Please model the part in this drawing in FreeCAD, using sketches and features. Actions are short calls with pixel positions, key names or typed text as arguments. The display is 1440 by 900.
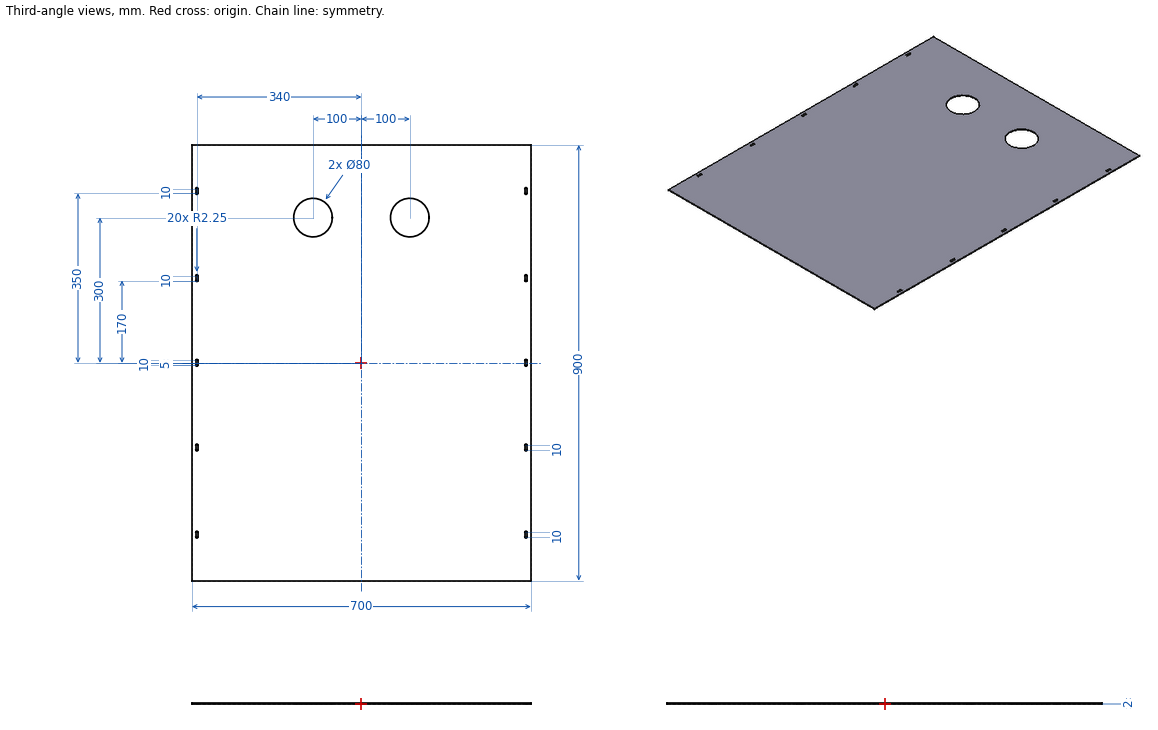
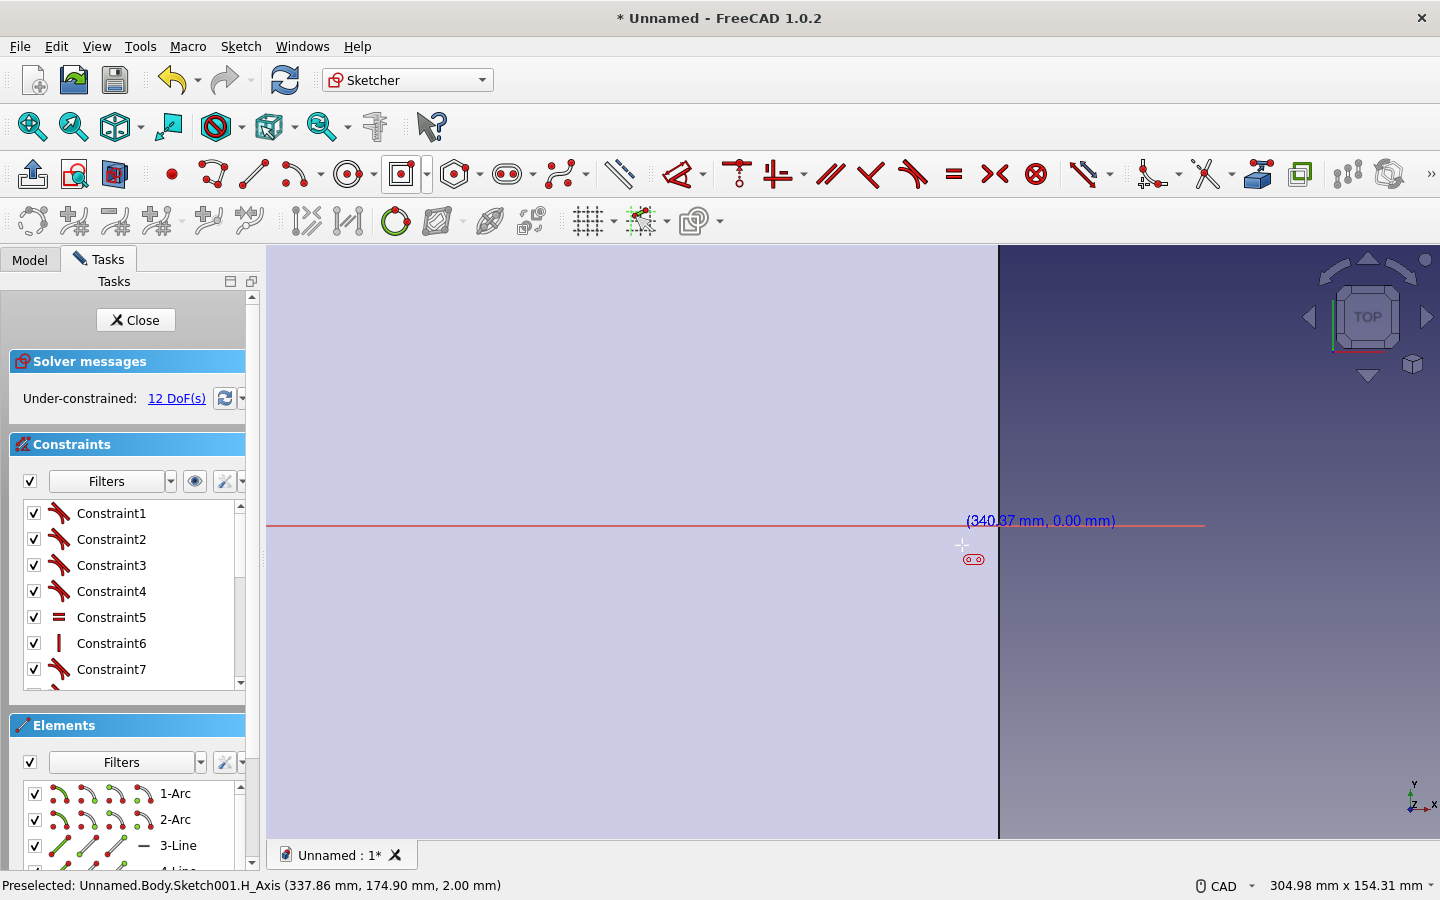
click(961, 545)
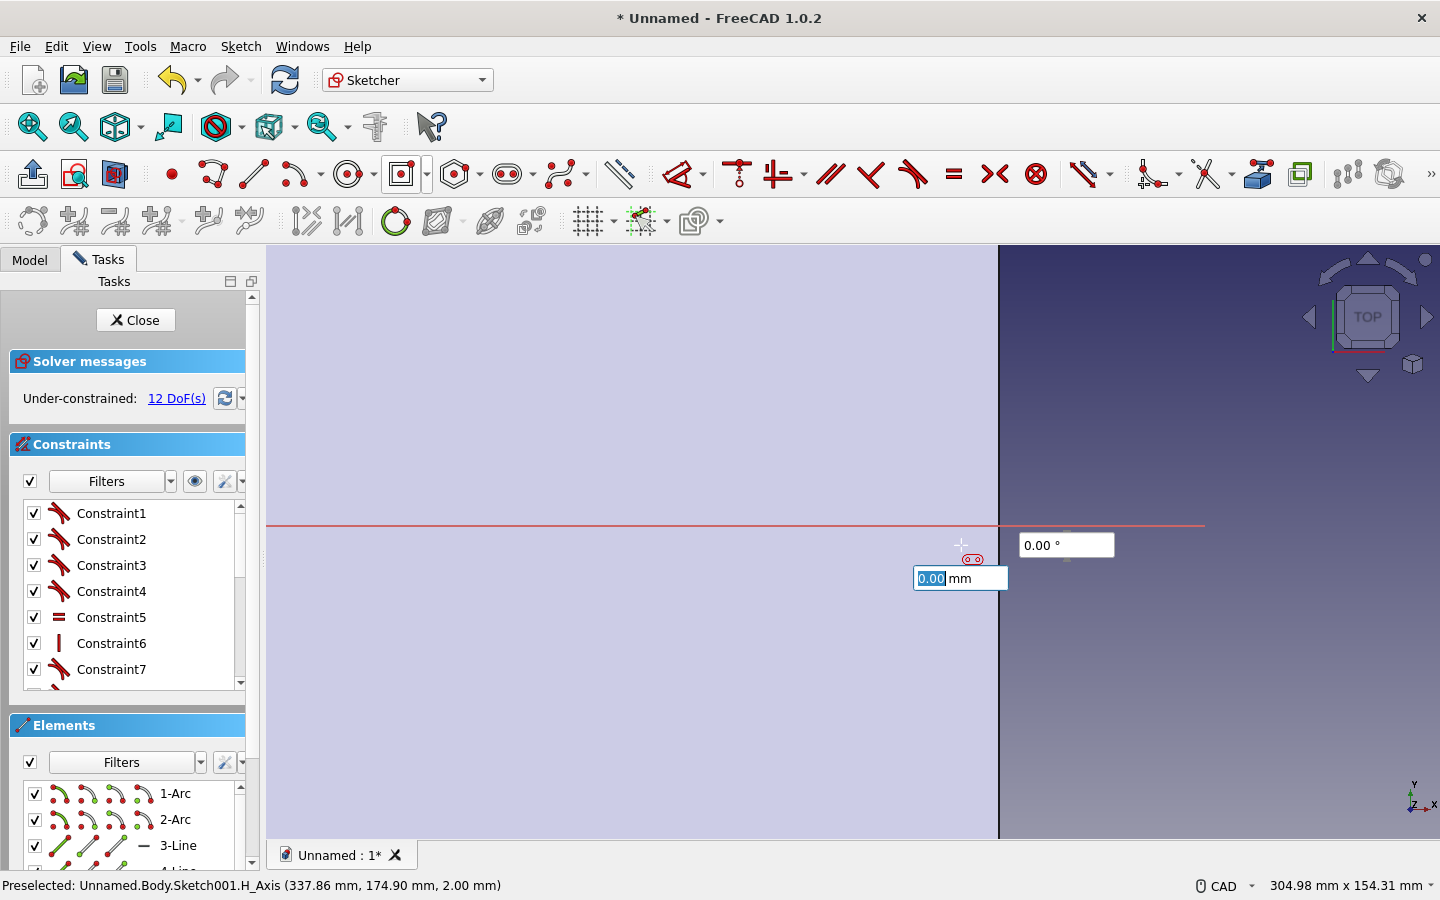
click(961, 506)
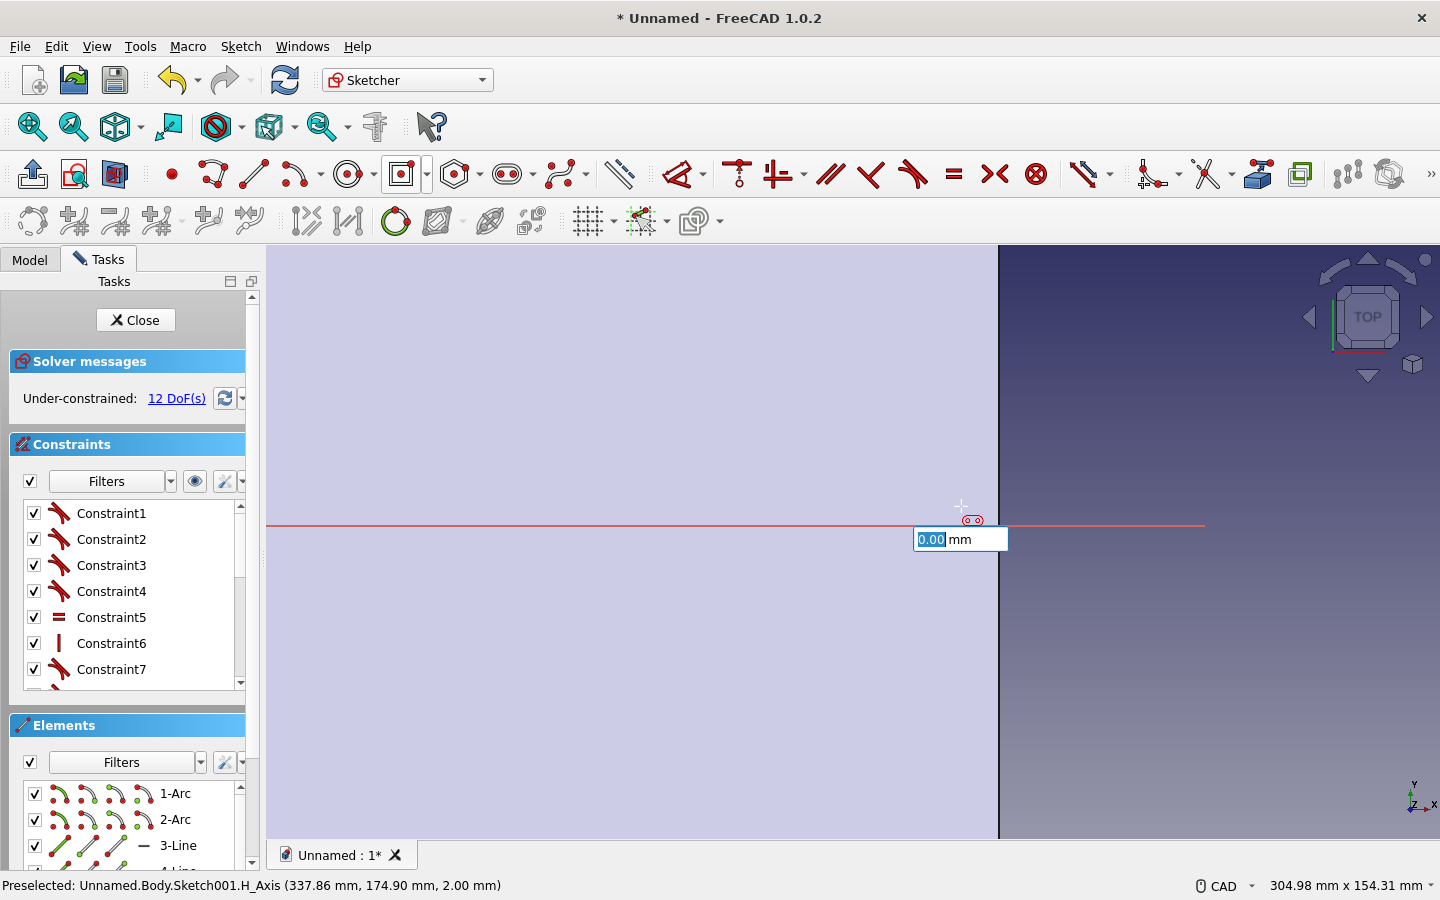
scroll(970, 531, up, 6)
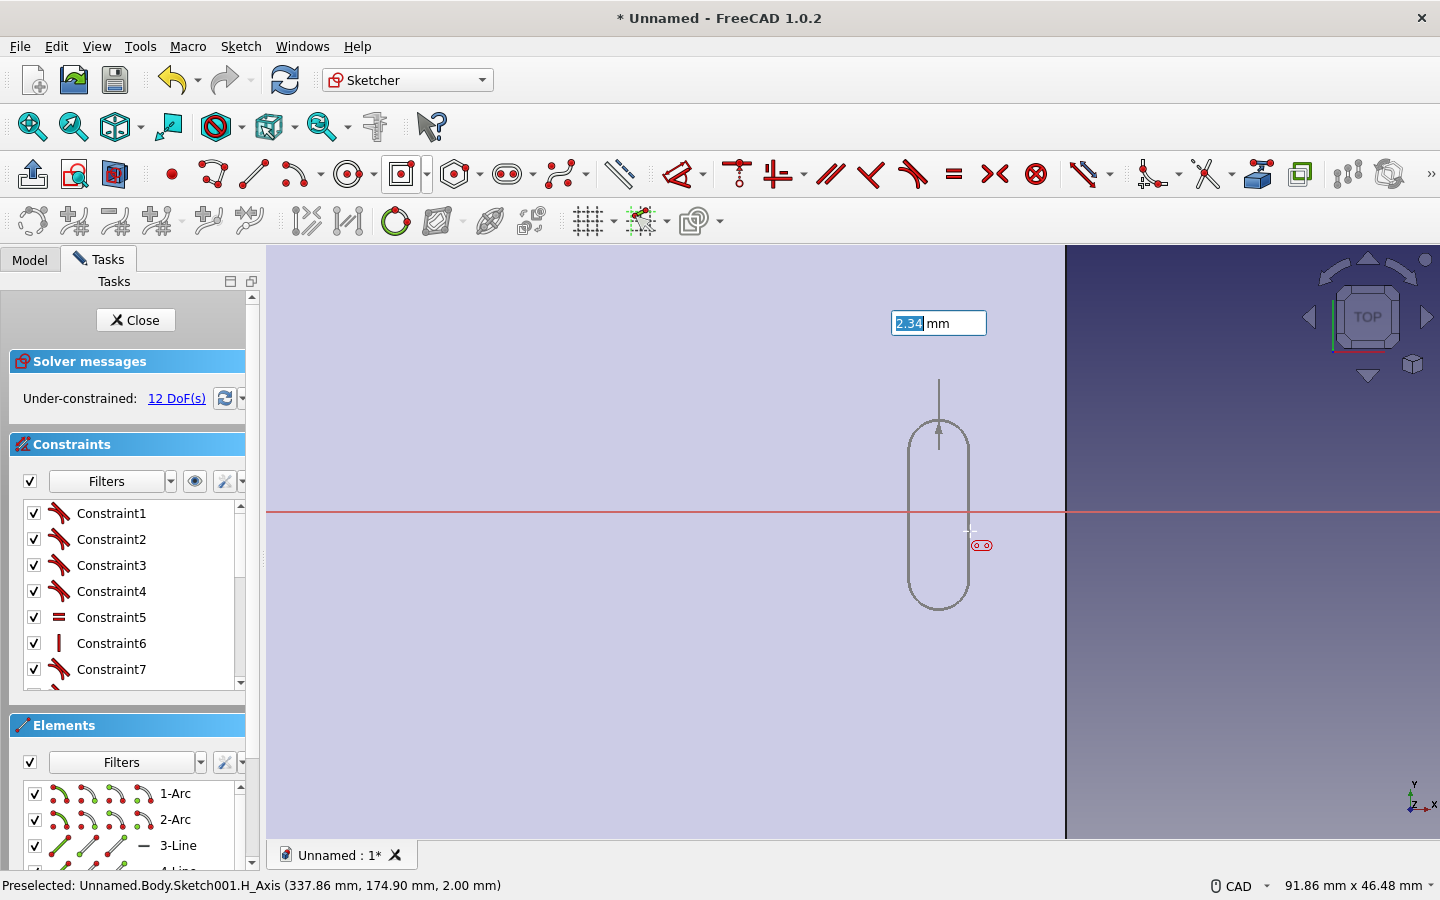
click(967, 531)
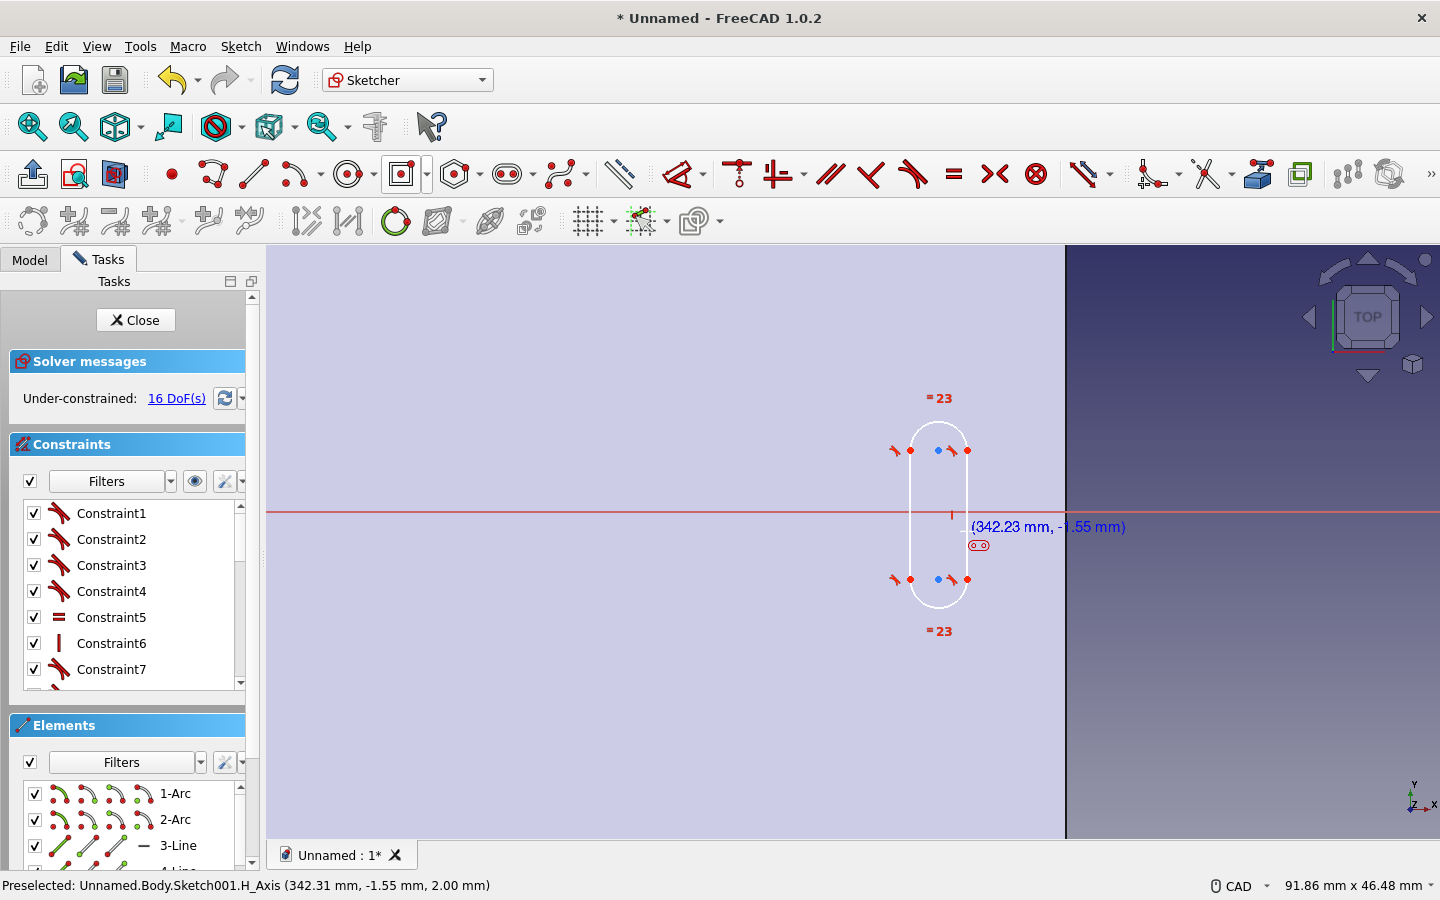
scroll(1004, 544, down, 15)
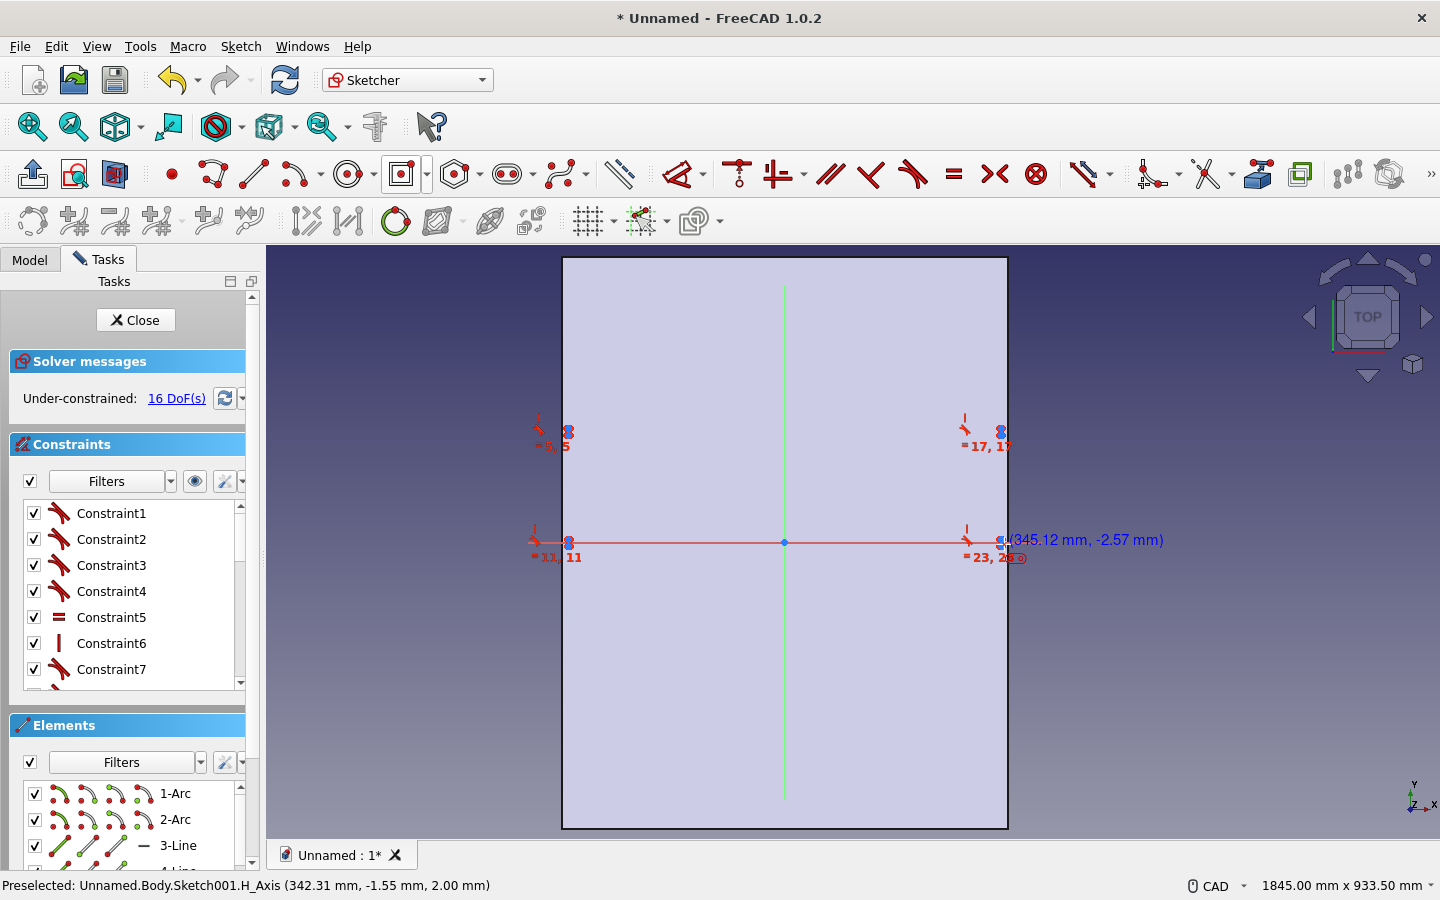
scroll(569, 320, up, 14)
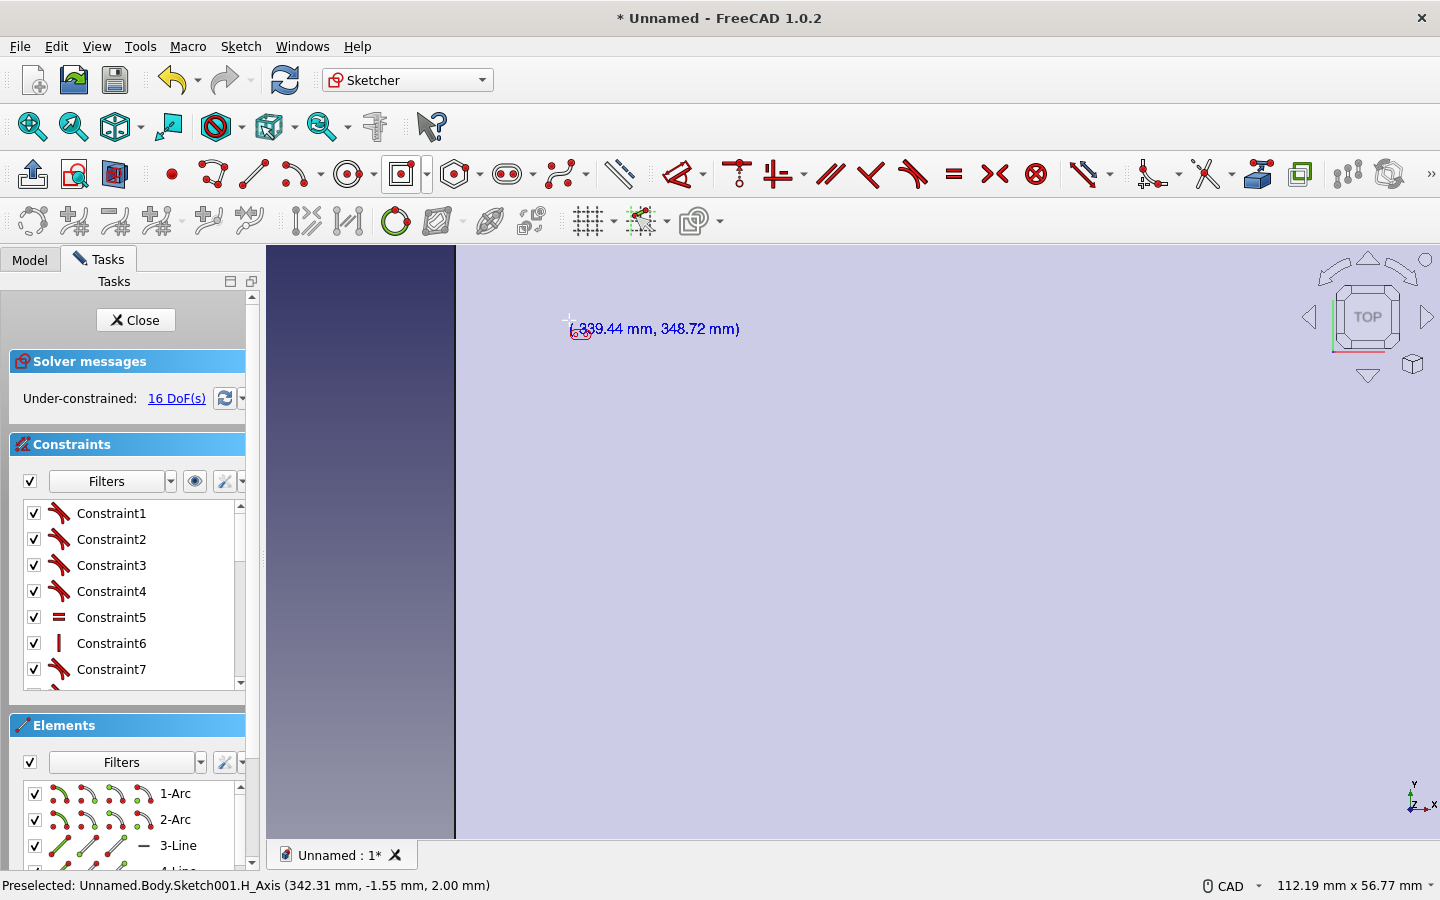
scroll(610, 362, down, 15)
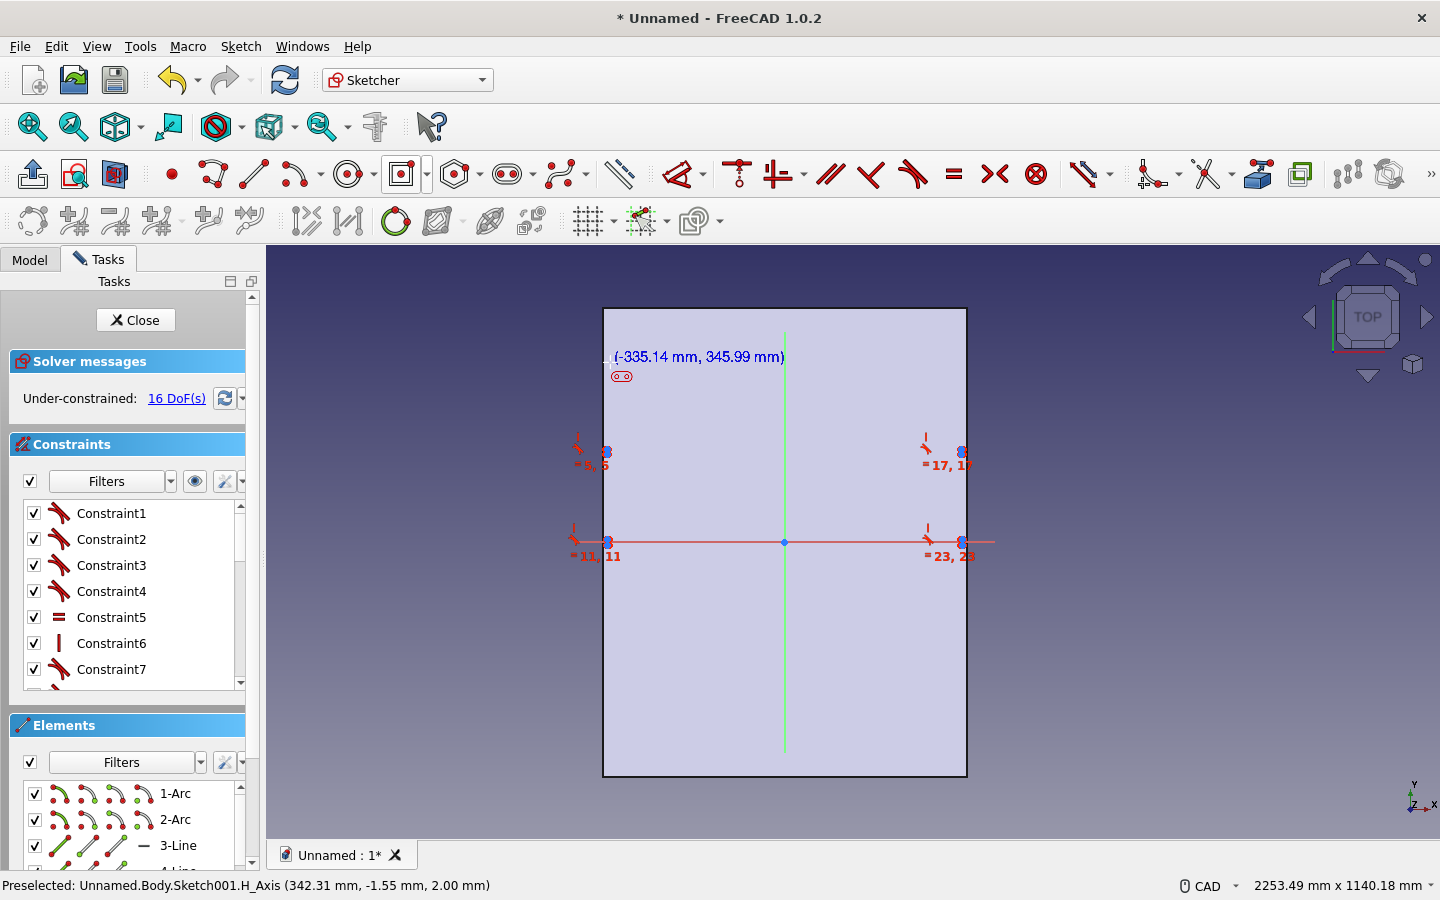
click(608, 360)